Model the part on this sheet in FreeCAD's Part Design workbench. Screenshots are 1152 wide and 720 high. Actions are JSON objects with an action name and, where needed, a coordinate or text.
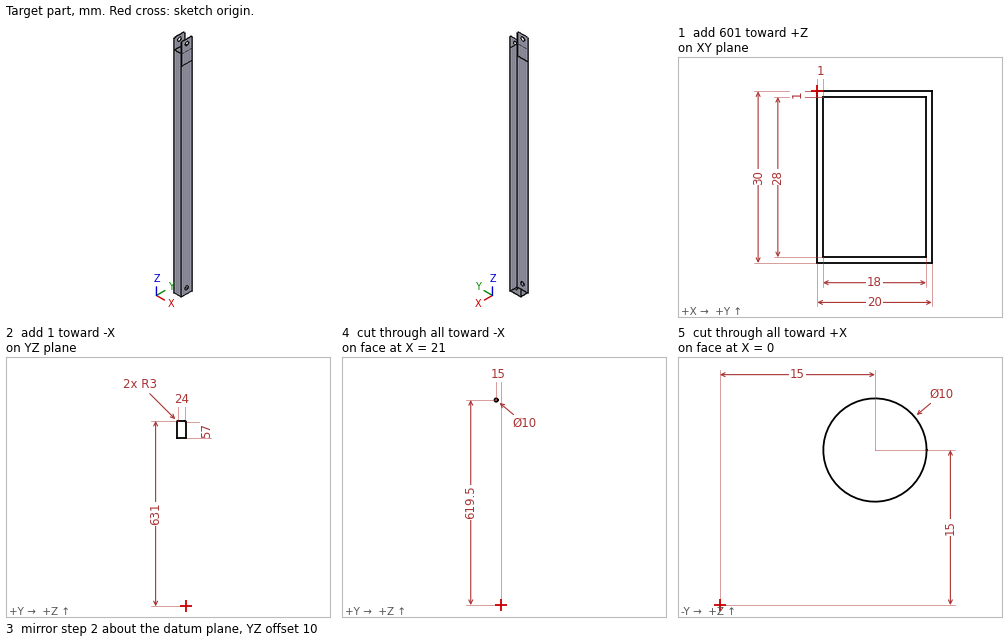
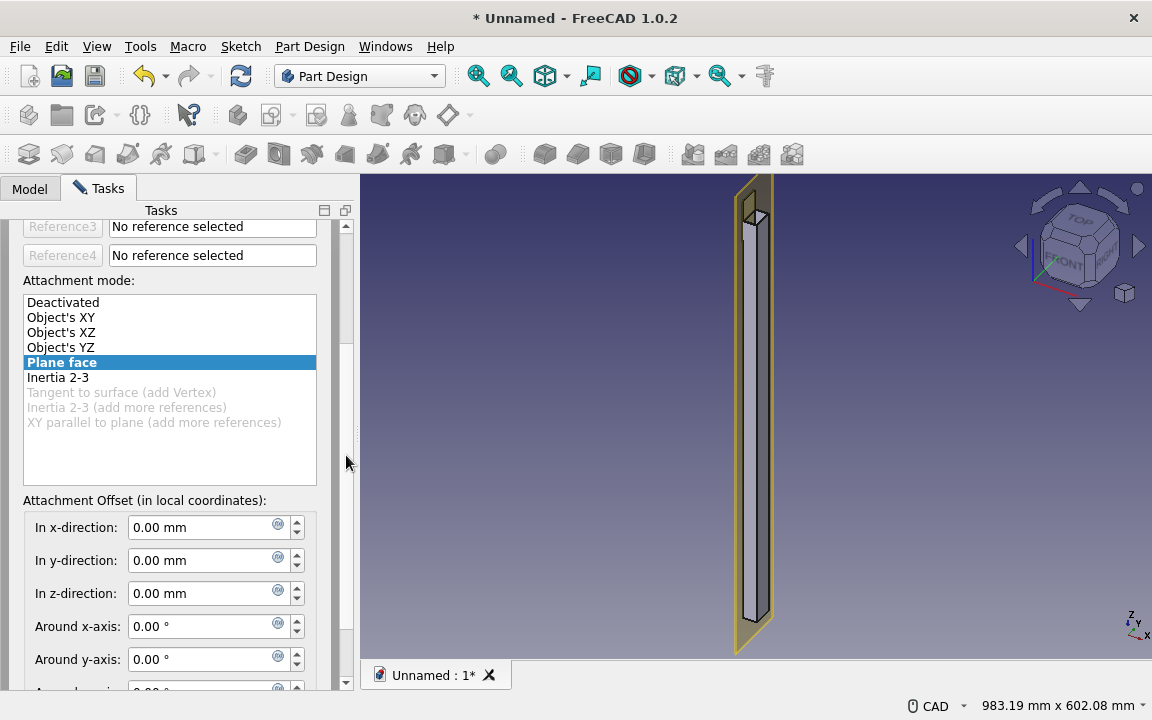
{"action": "triple_click", "coordinate": [210, 594]}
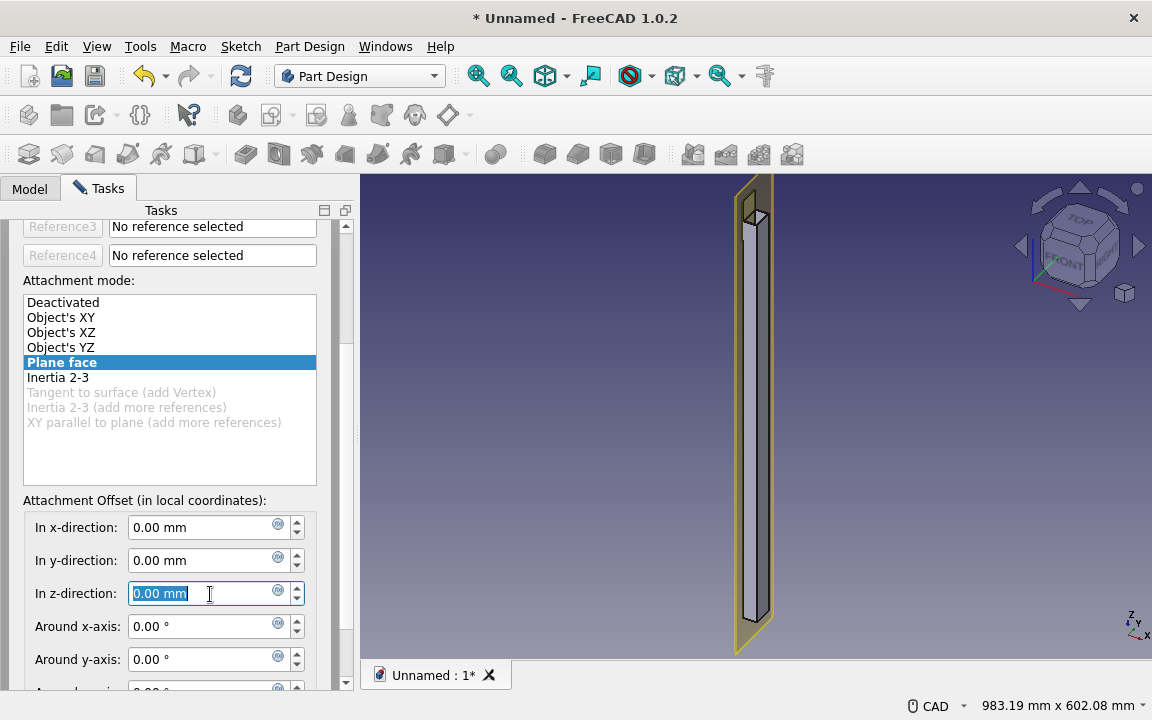
{"action": "type", "text": "10"}
{"action": "key", "text": "Tab"}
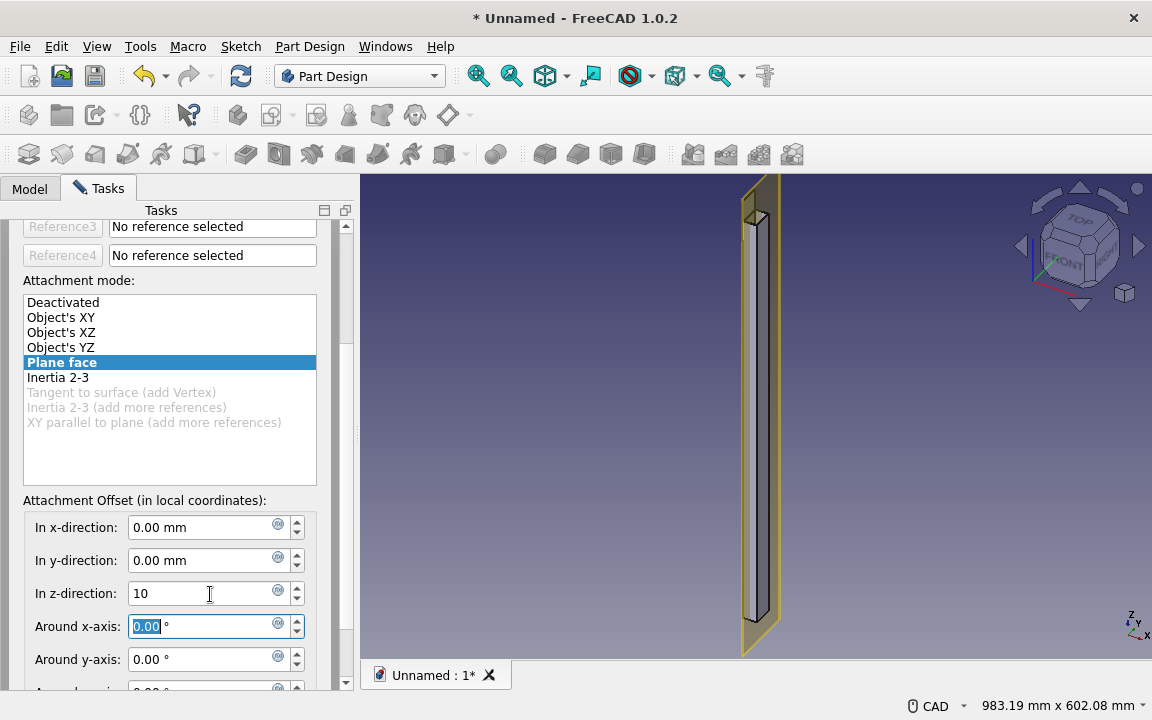
{"action": "scroll", "coordinate": [346, 455], "scroll_direction": "up", "scroll_amount": 4}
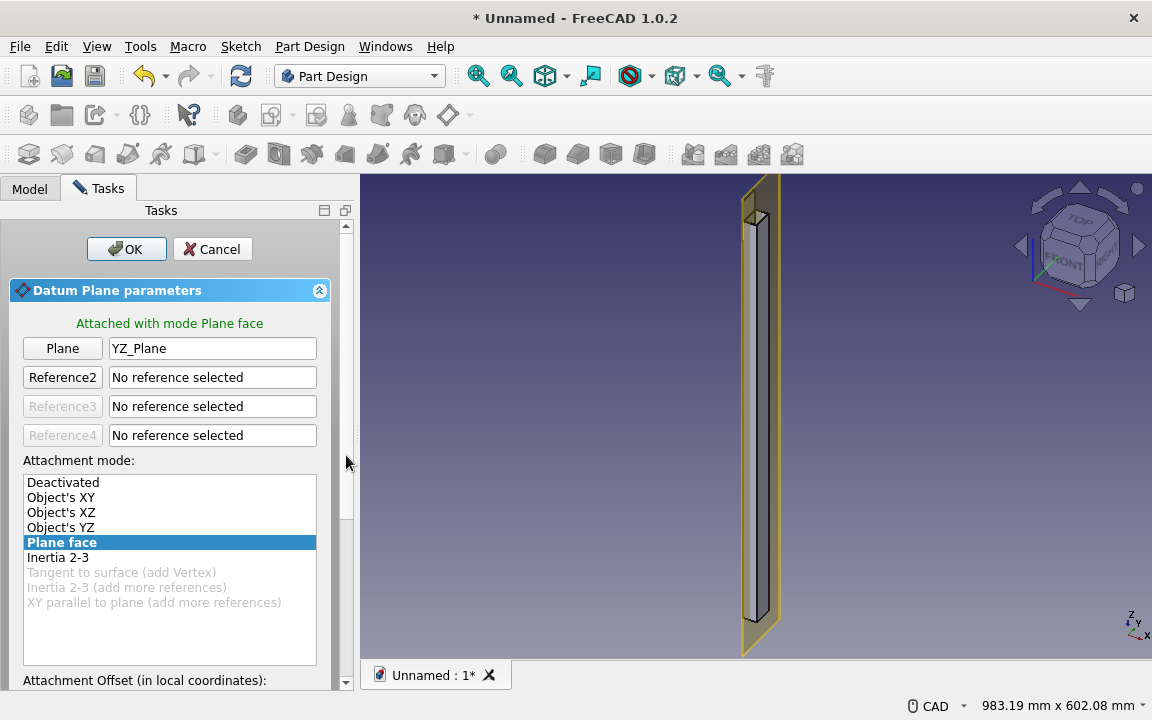
{"action": "left_click", "coordinate": [127, 249]}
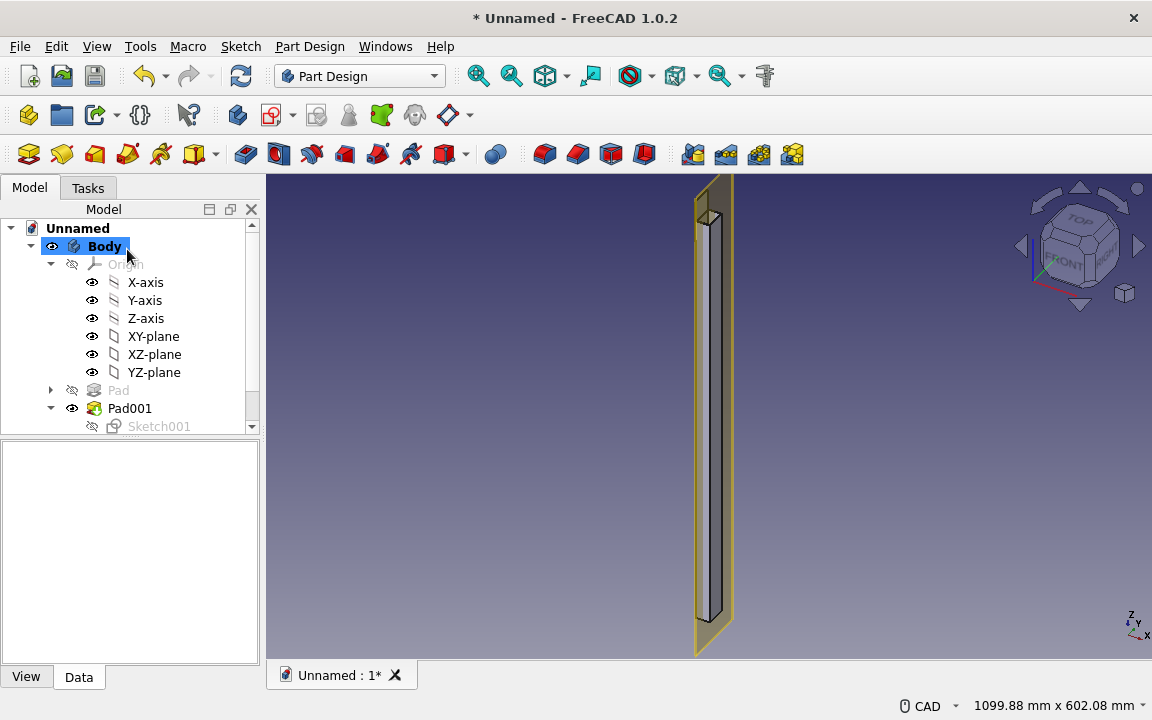
{"action": "left_click", "coordinate": [117, 408]}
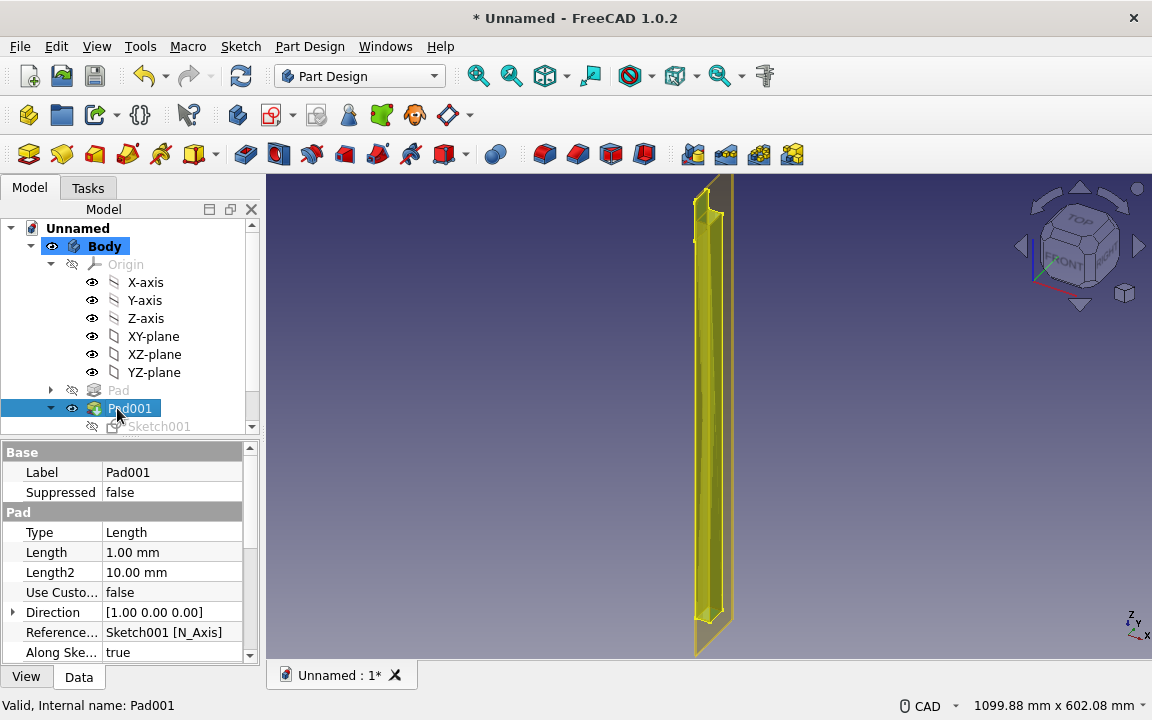
{"action": "left_click", "coordinate": [693, 154]}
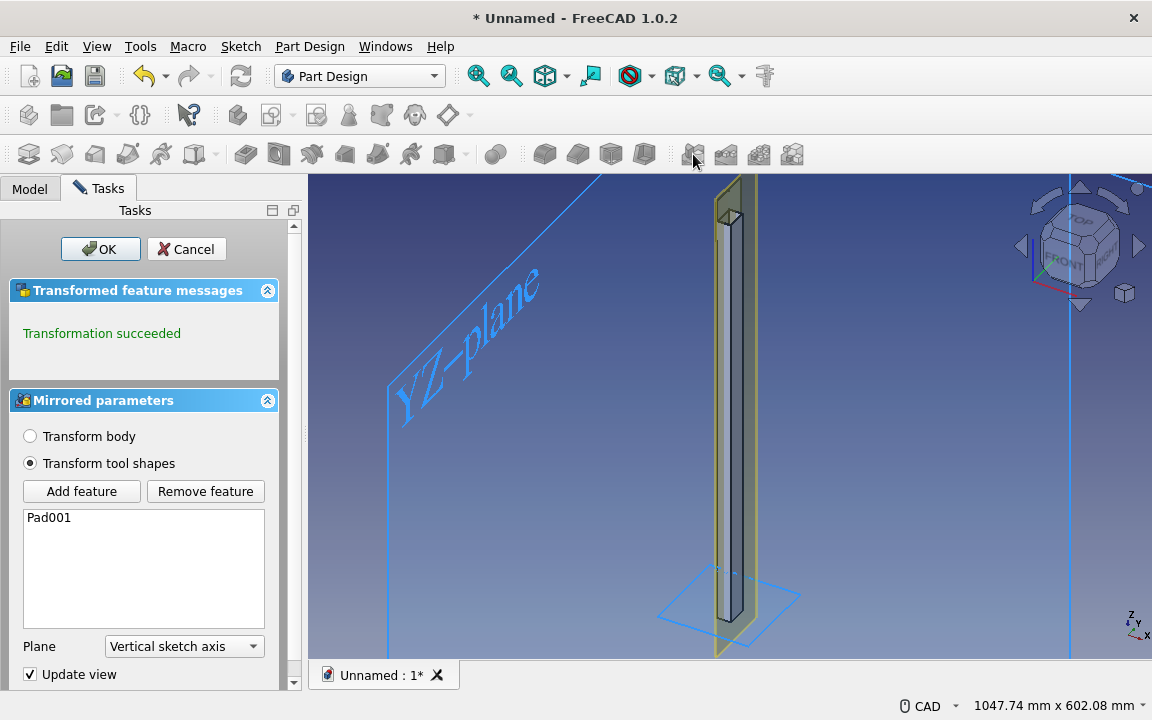
{"action": "left_click", "coordinate": [185, 646]}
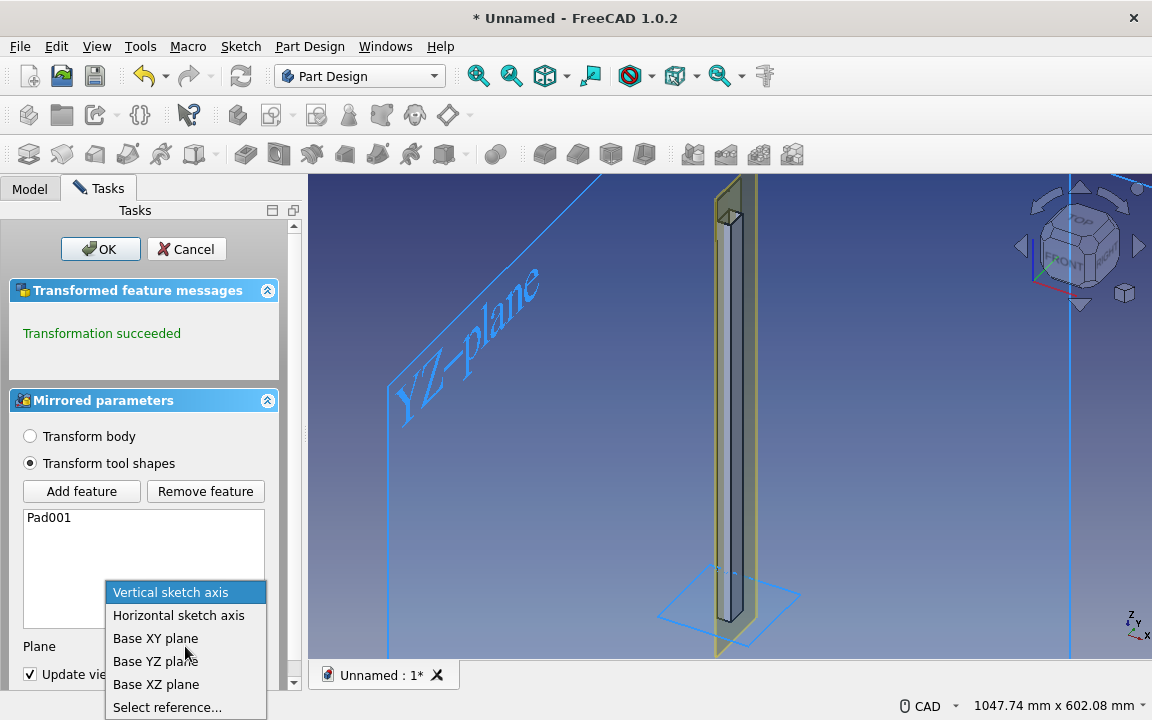
{"action": "left_click", "coordinate": [184, 708]}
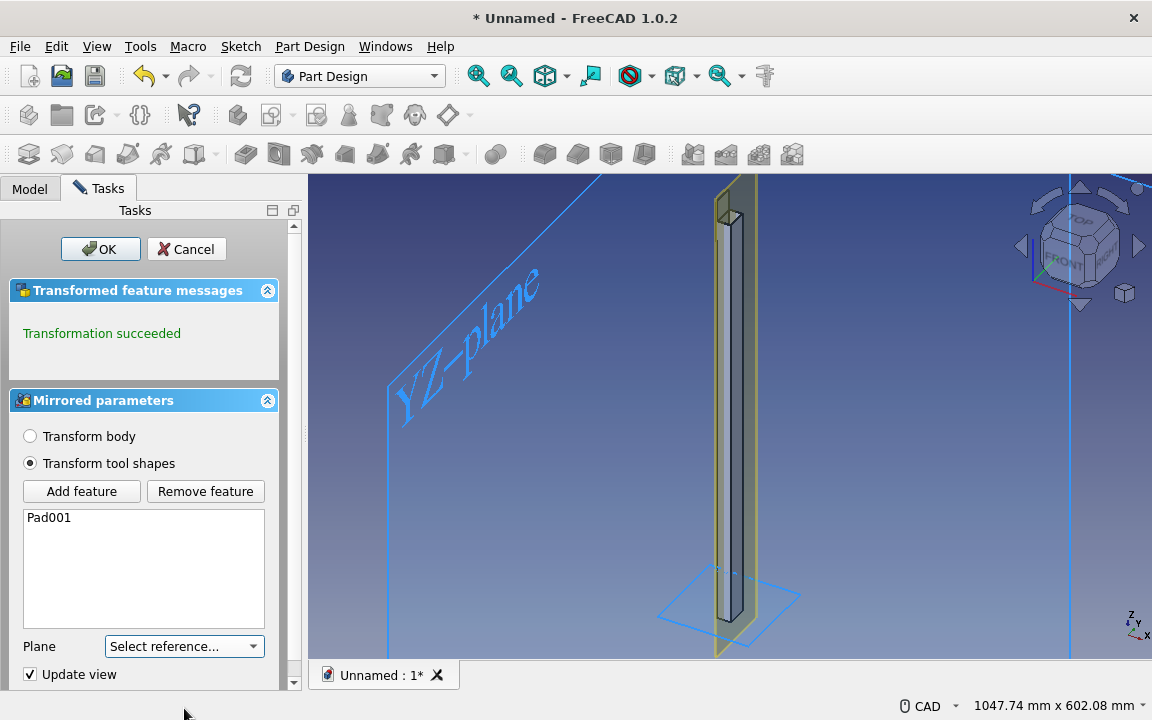
{"action": "left_click", "coordinate": [30, 188]}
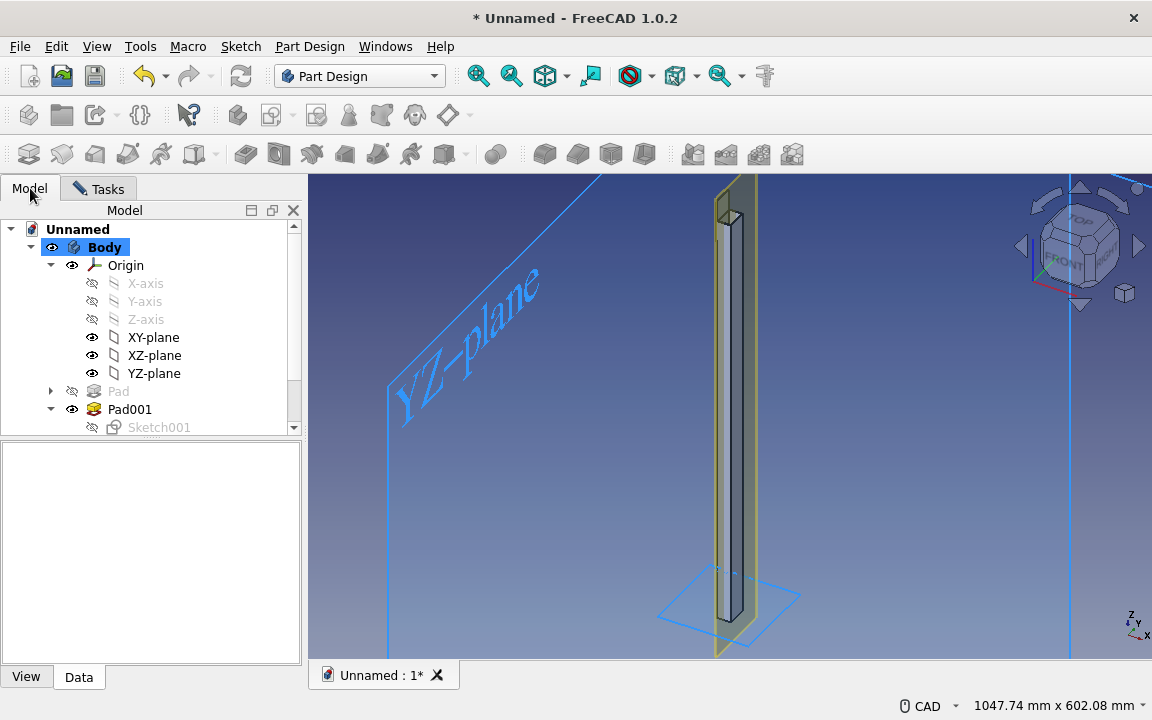
{"action": "scroll", "coordinate": [101, 333], "scroll_direction": "down", "scroll_amount": 3}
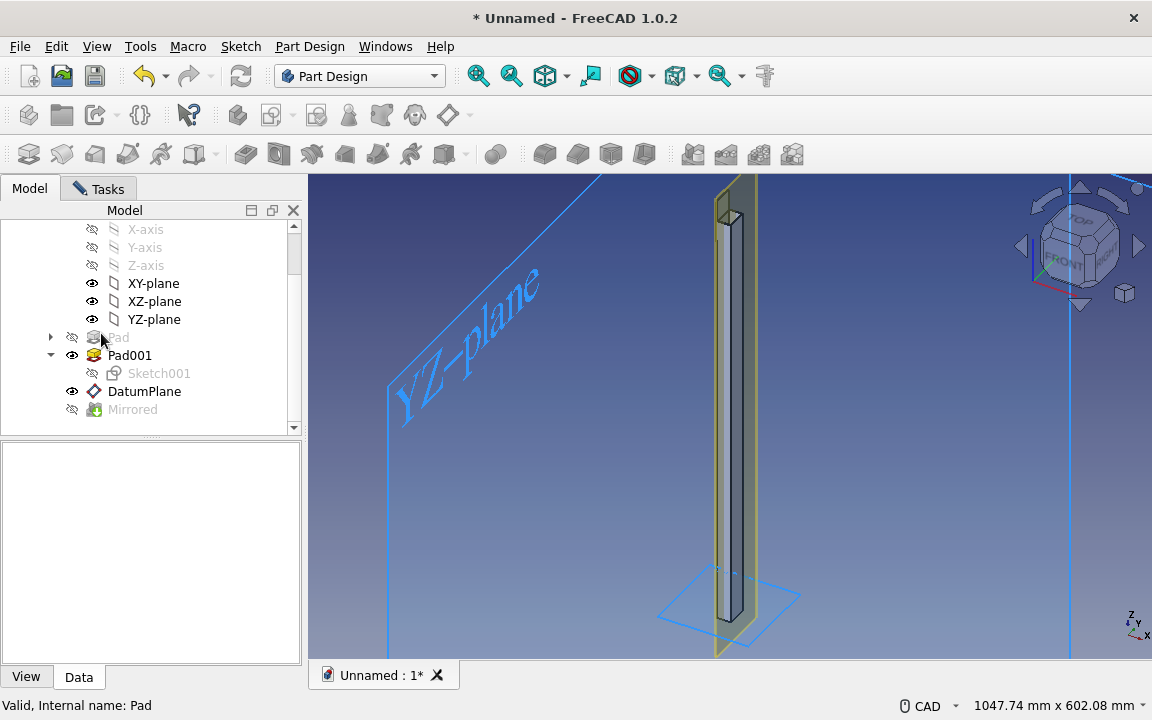
{"action": "left_click", "coordinate": [117, 391]}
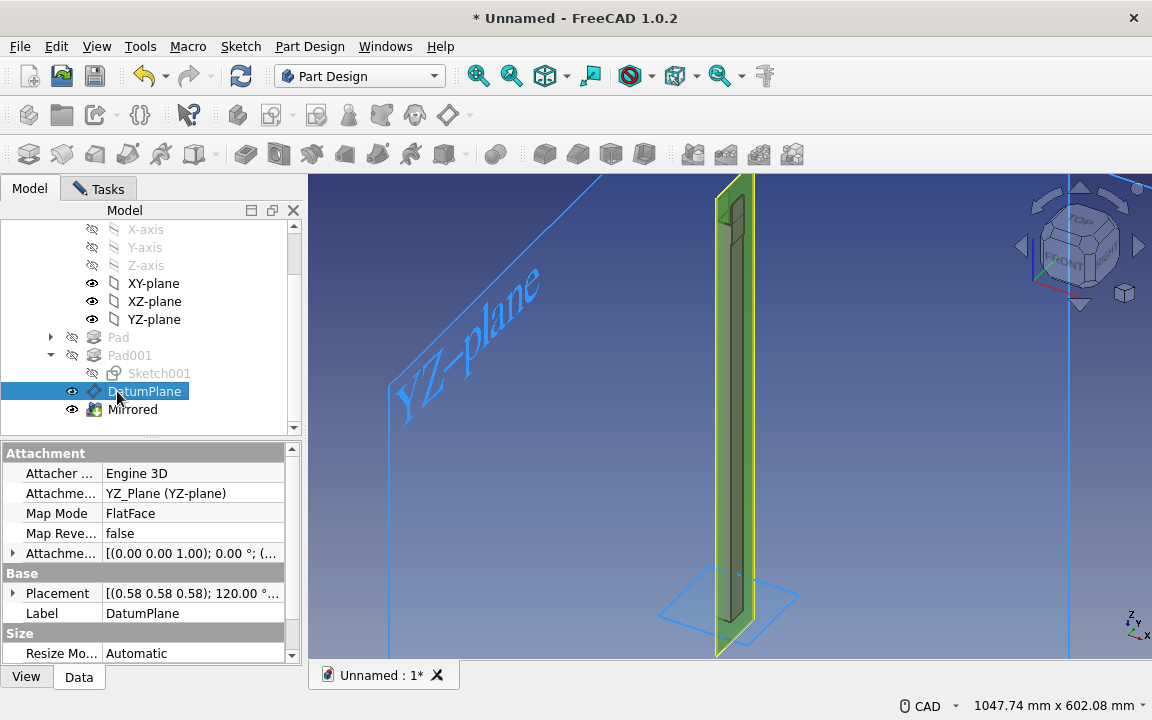
{"action": "left_click", "coordinate": [98, 188]}